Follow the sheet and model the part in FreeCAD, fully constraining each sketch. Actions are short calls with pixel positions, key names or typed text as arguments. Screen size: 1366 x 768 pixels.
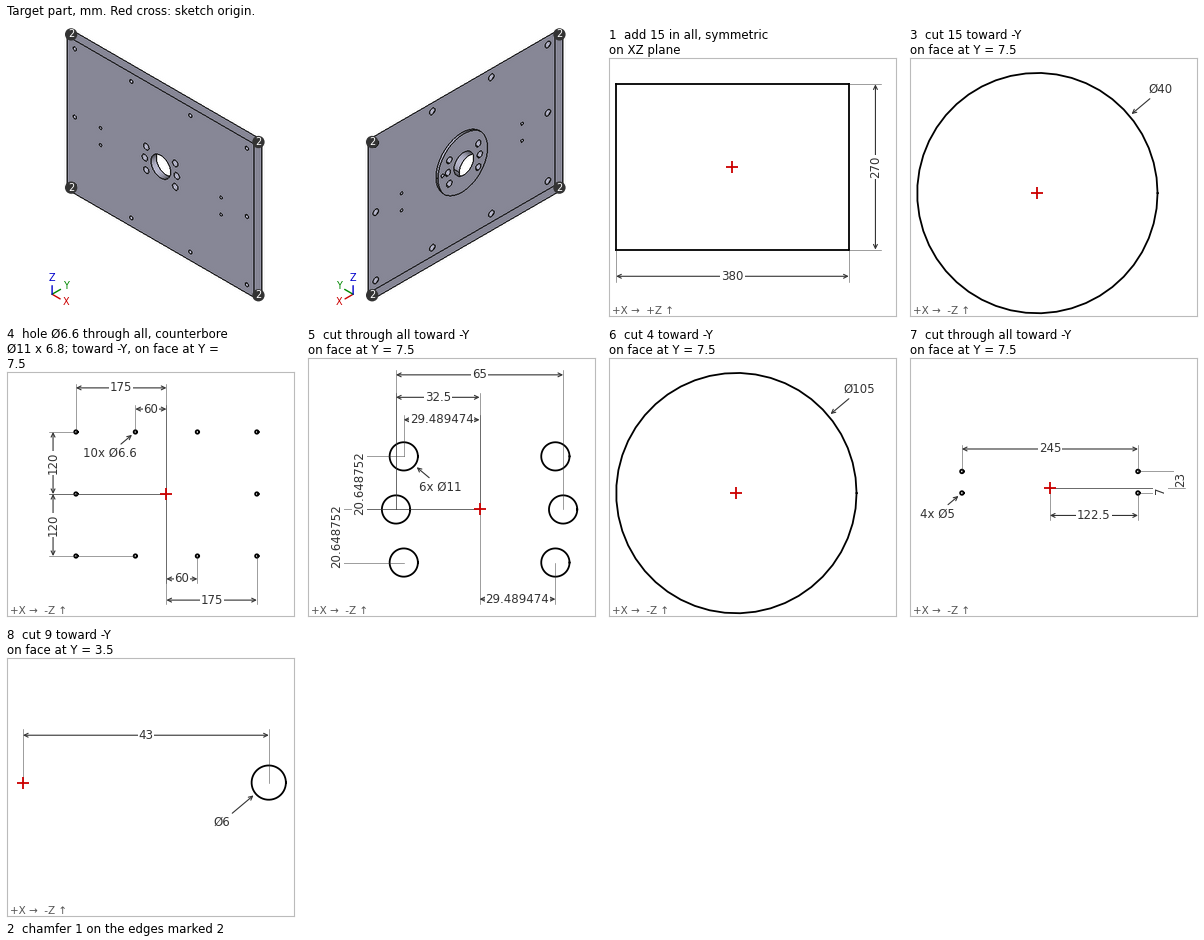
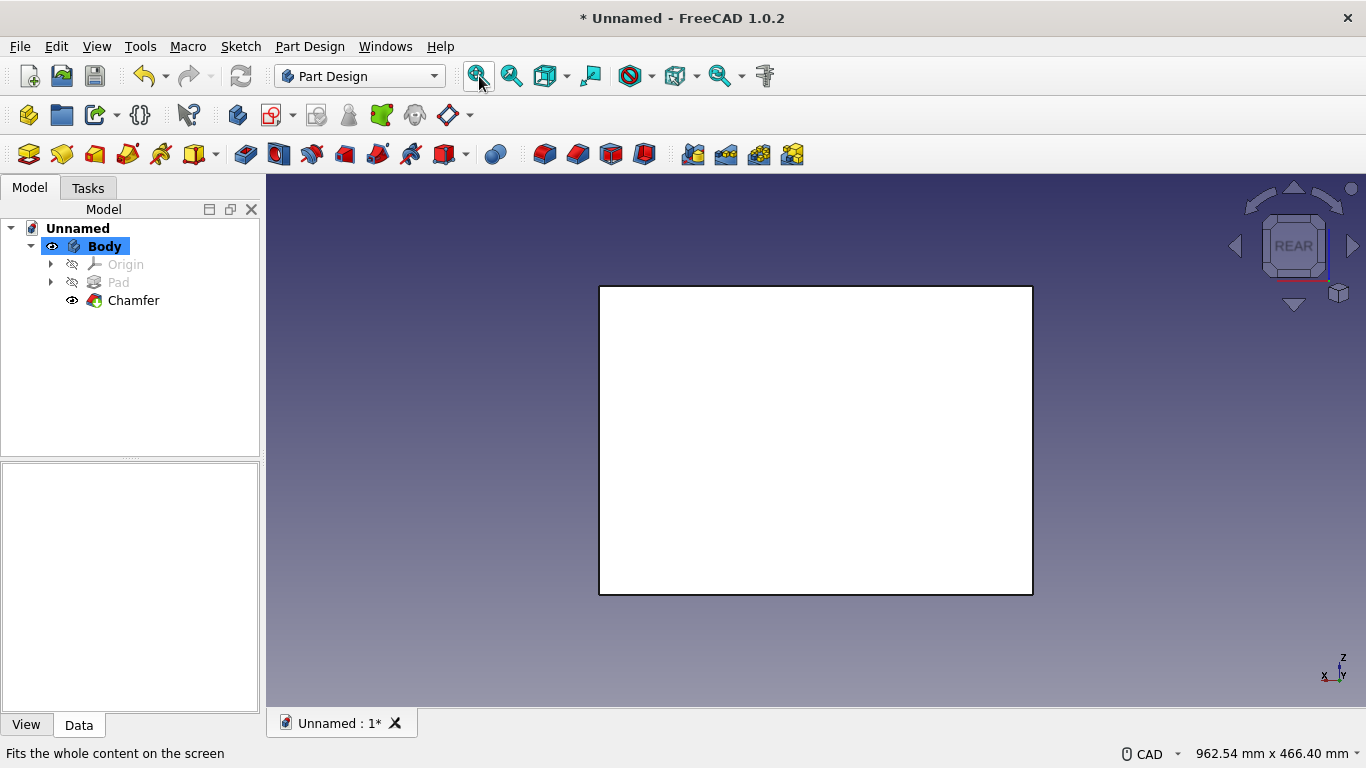
click(754, 439)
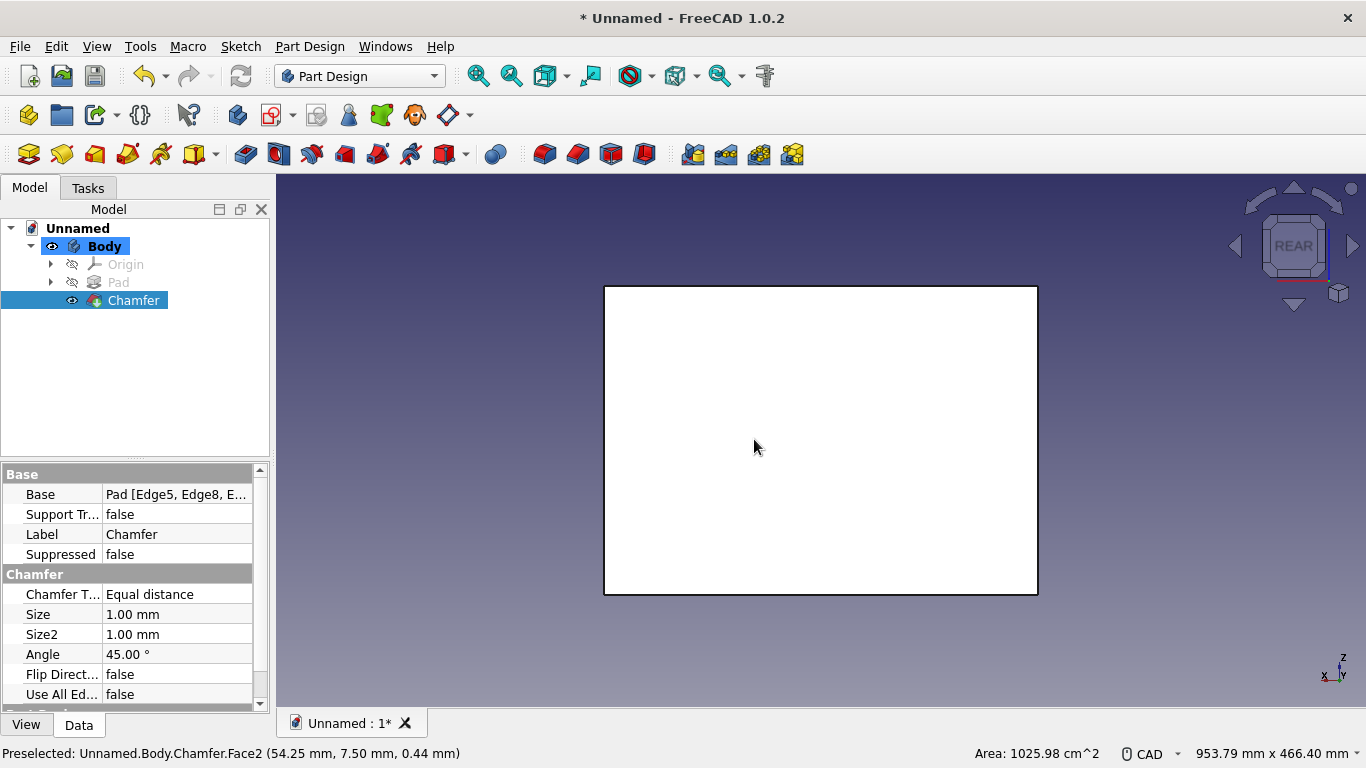
click(270, 116)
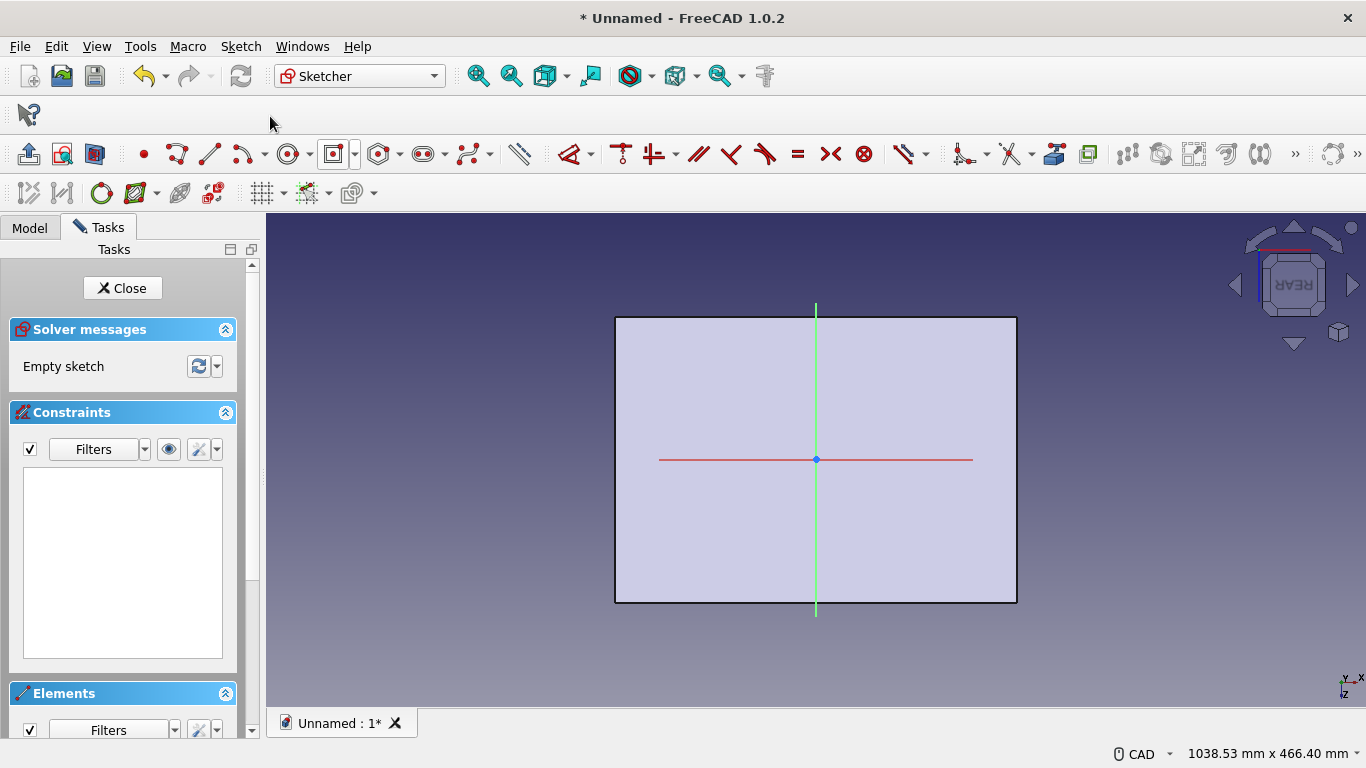
scroll(827, 460, up, 10)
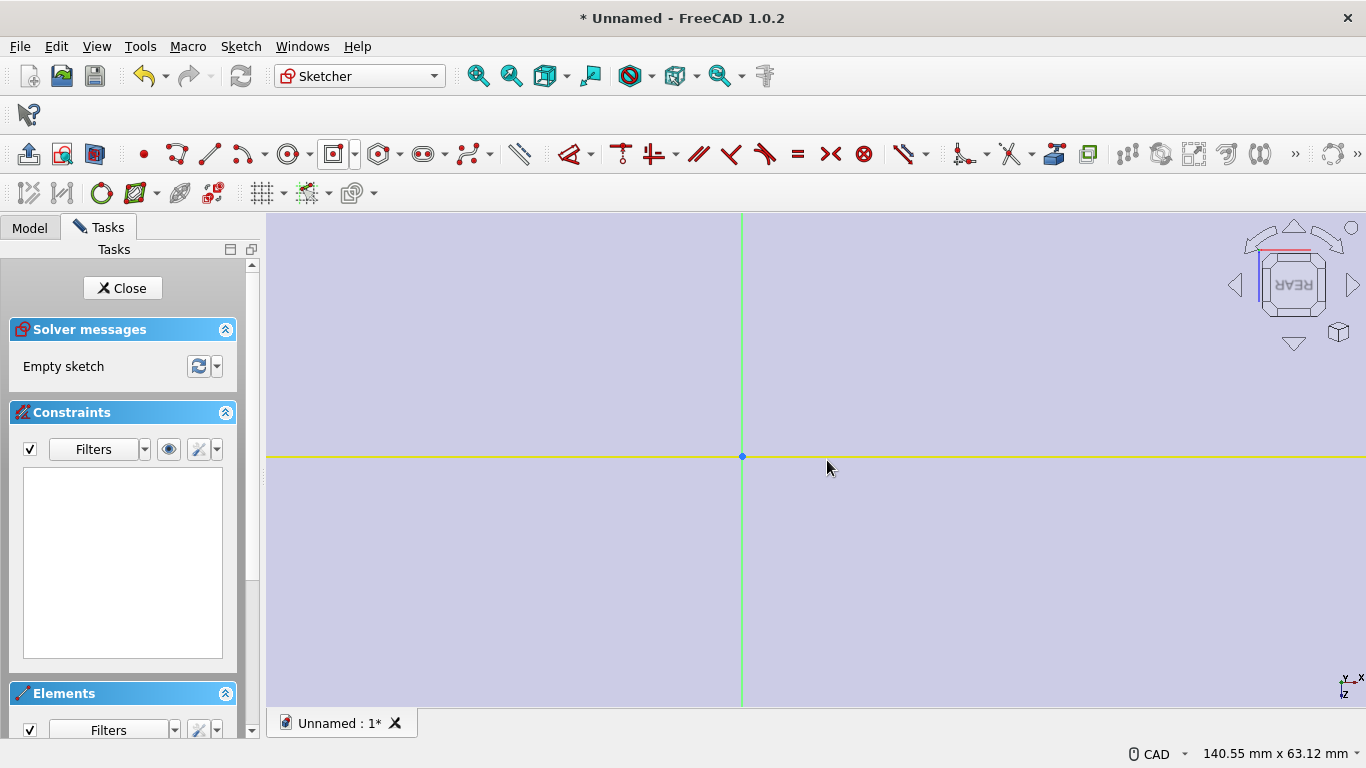
click(288, 154)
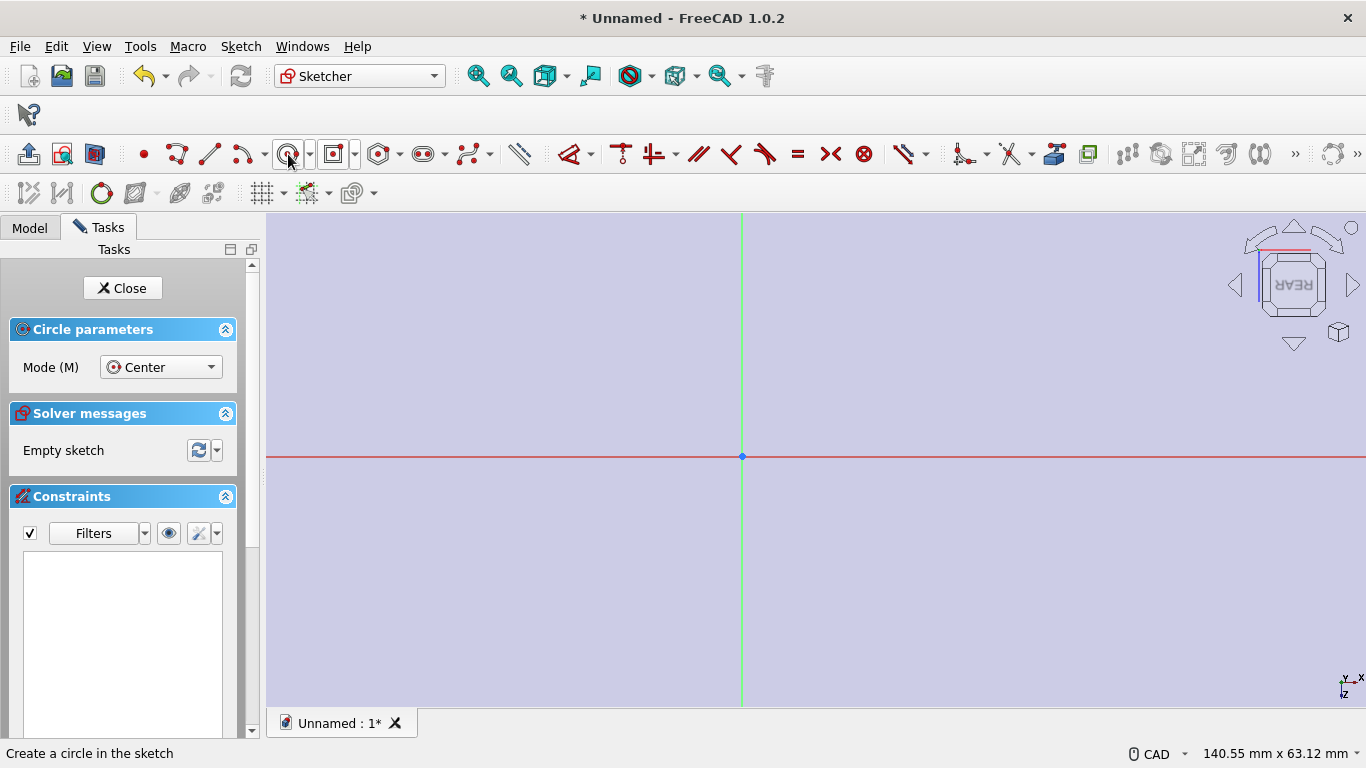
click(742, 457)
click(853, 346)
key(Escape)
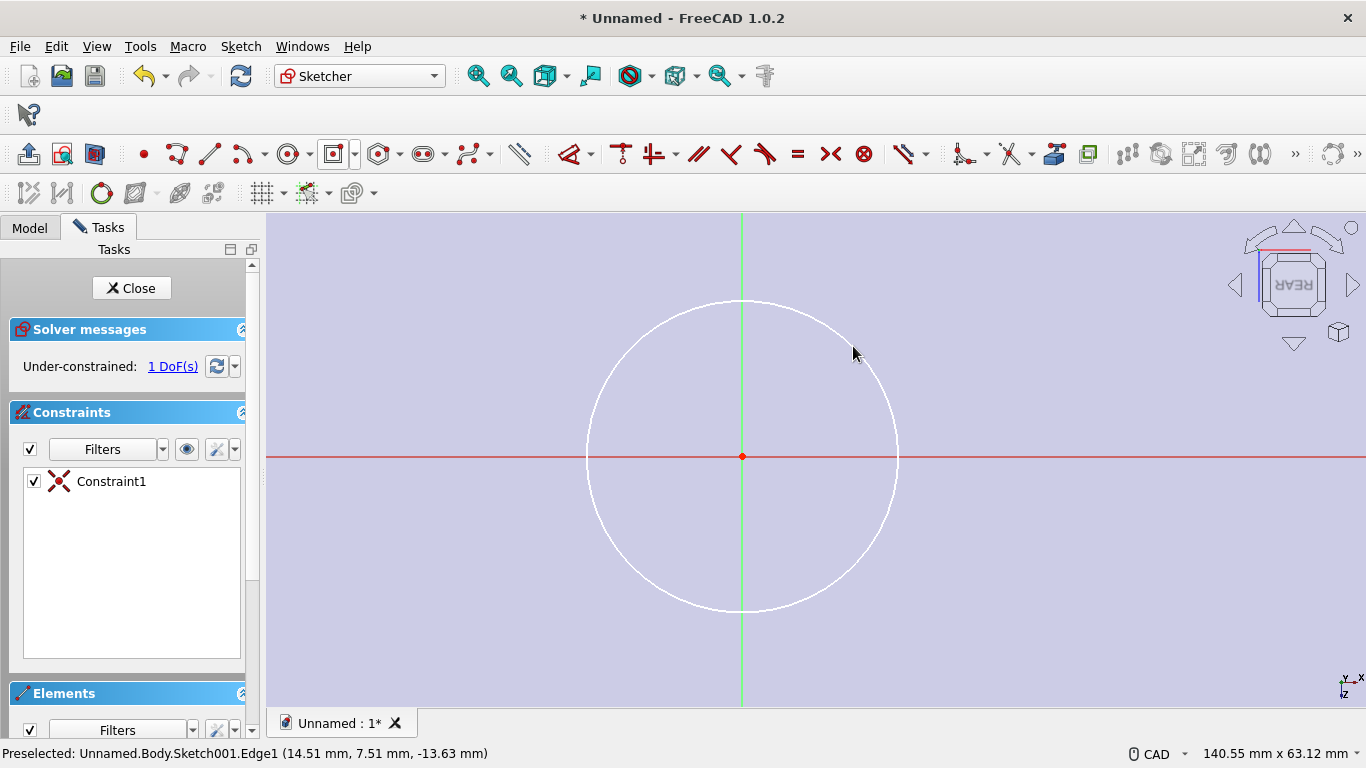
click(568, 154)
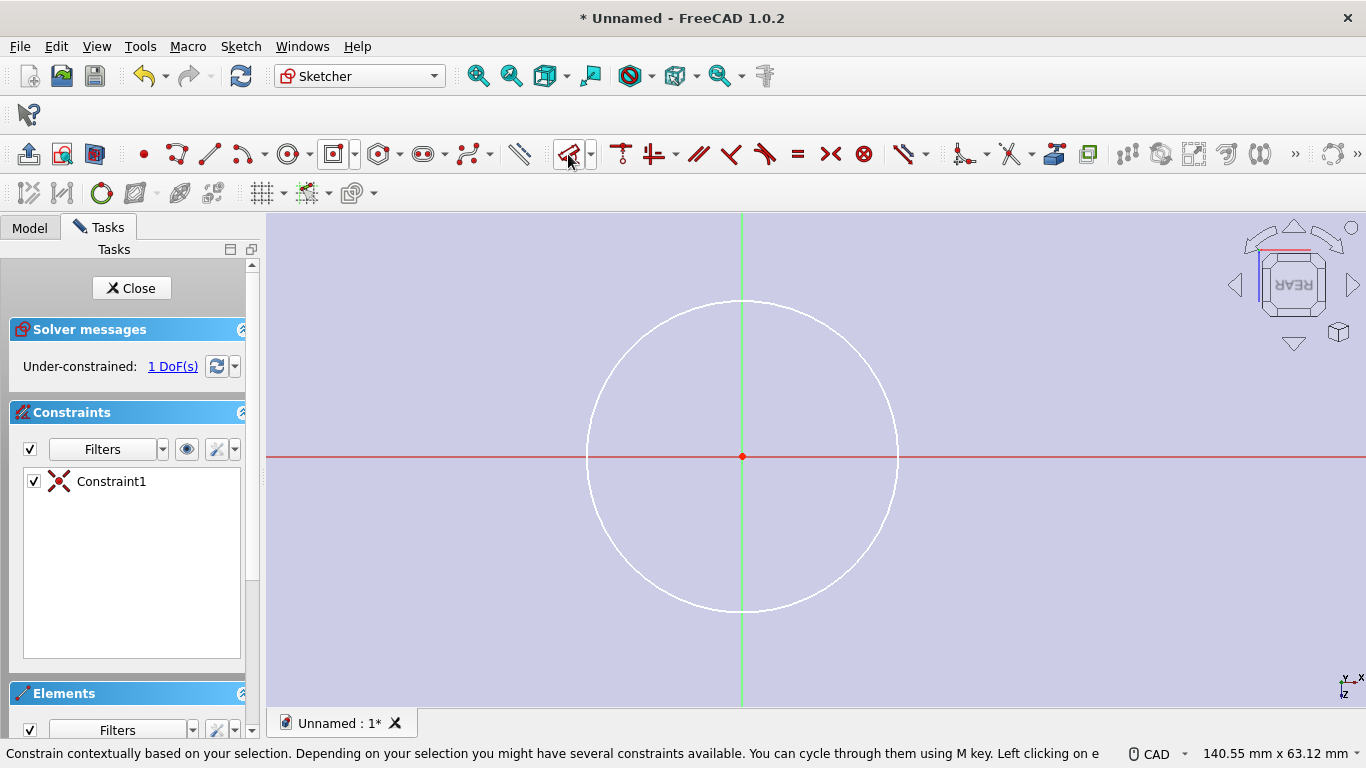
click(852, 346)
click(874, 323)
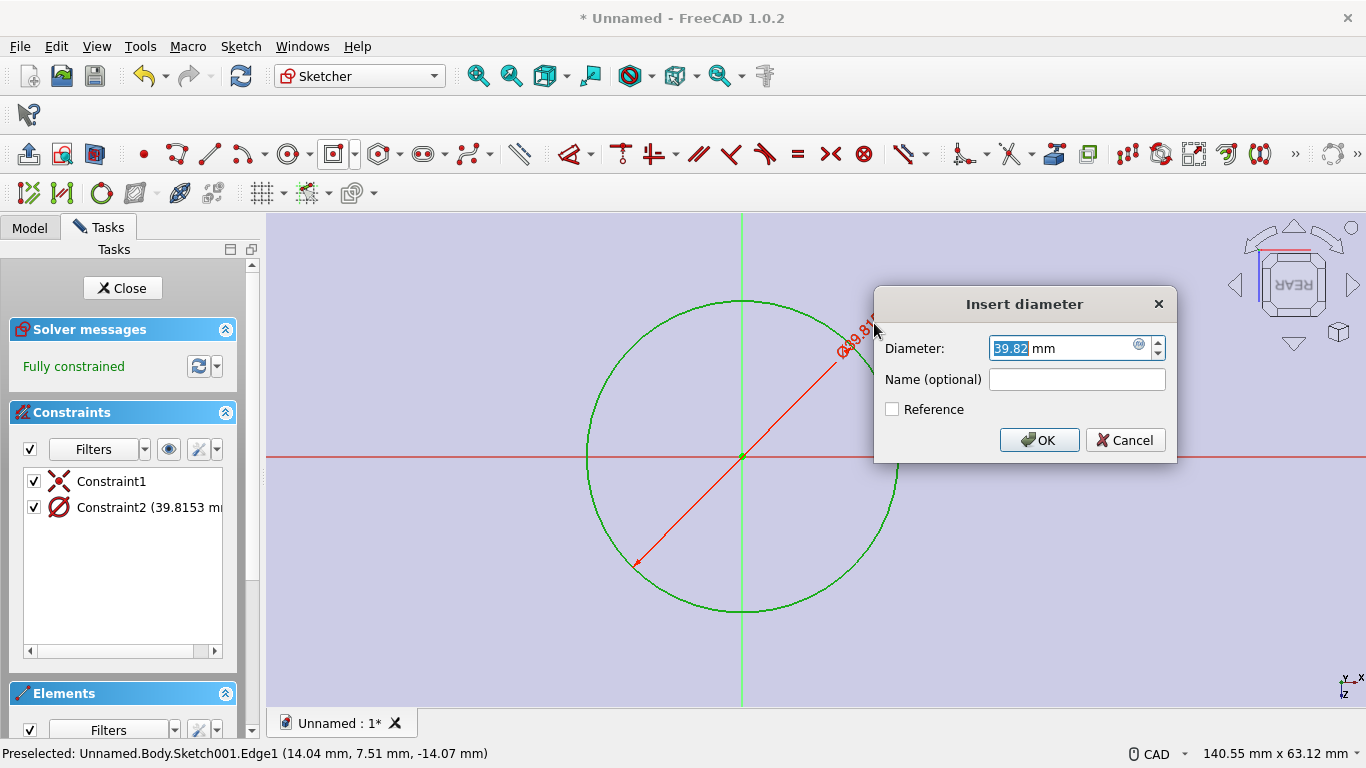
text(40)
key(Return)
key(Escape)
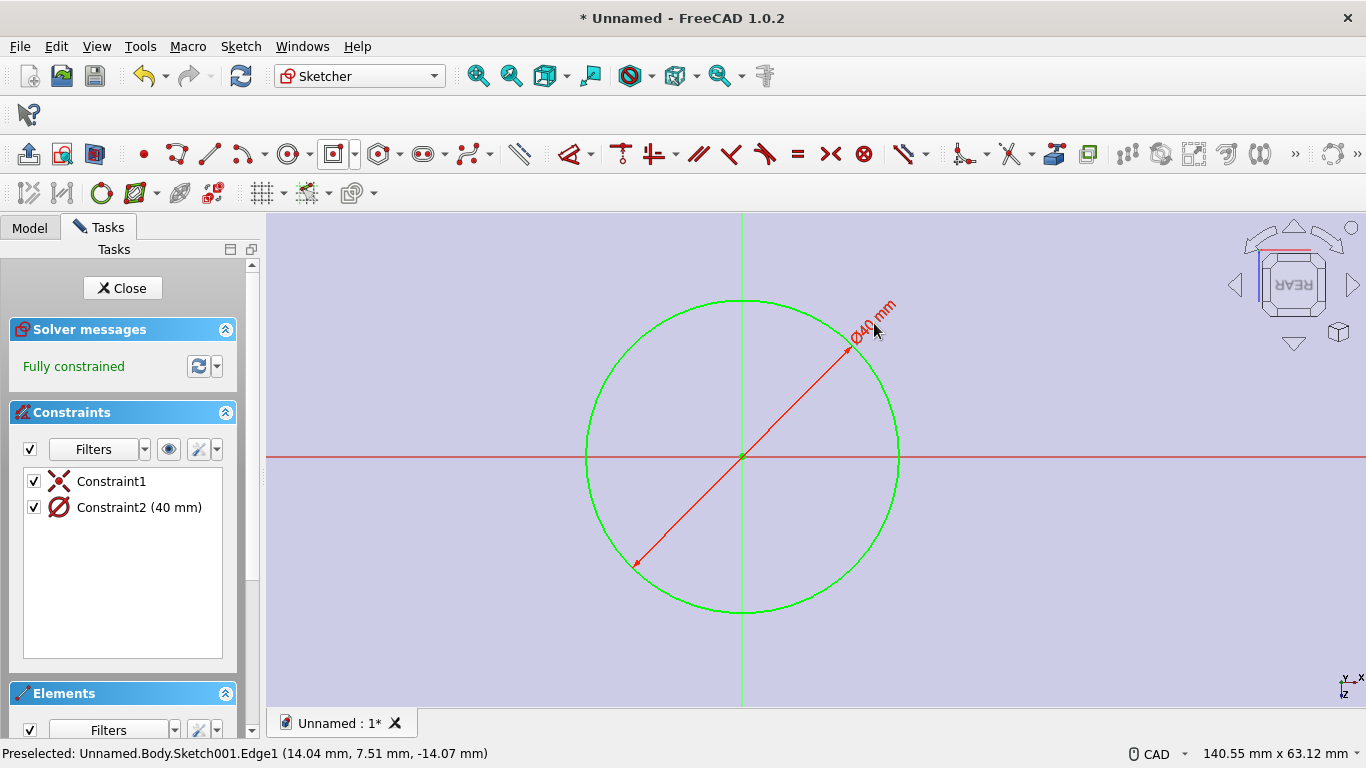
click(123, 288)